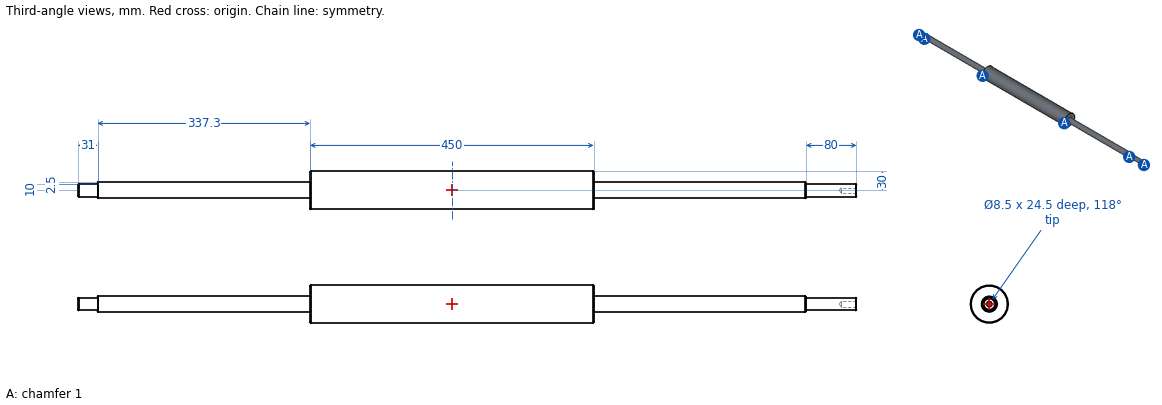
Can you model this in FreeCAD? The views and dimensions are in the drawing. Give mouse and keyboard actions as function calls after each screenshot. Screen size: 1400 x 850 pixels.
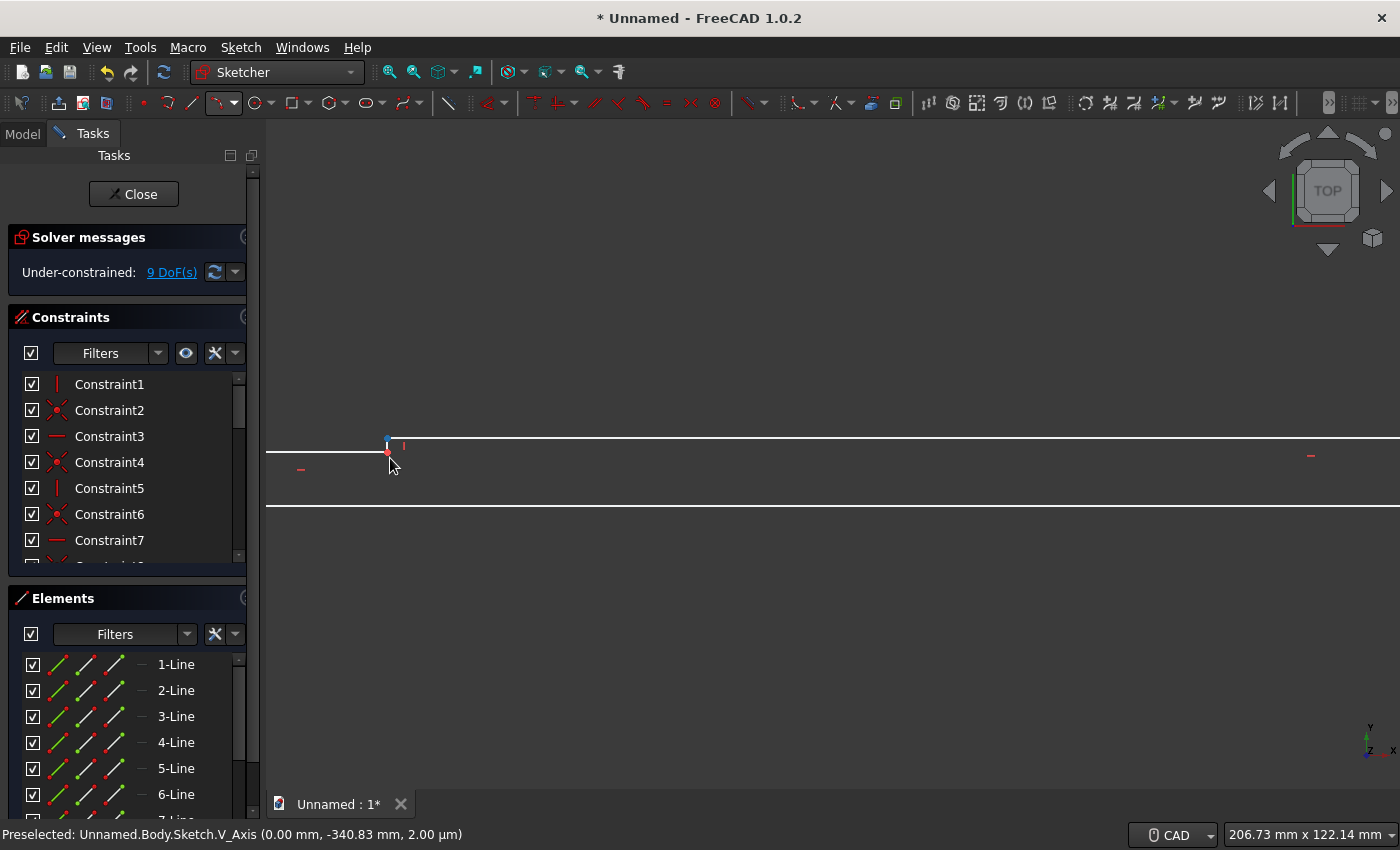
click(387, 452)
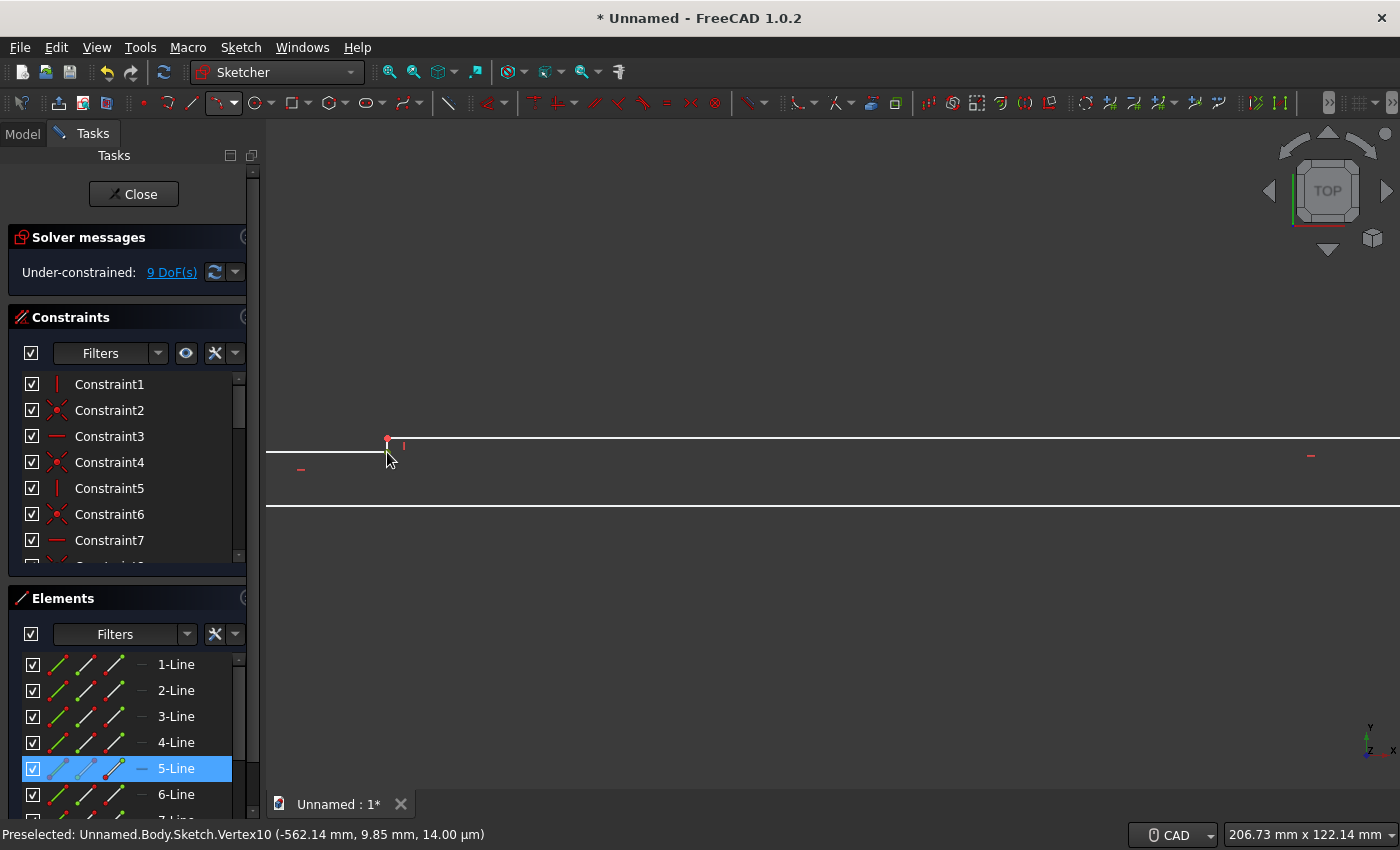
scroll(481, 457, down, 12)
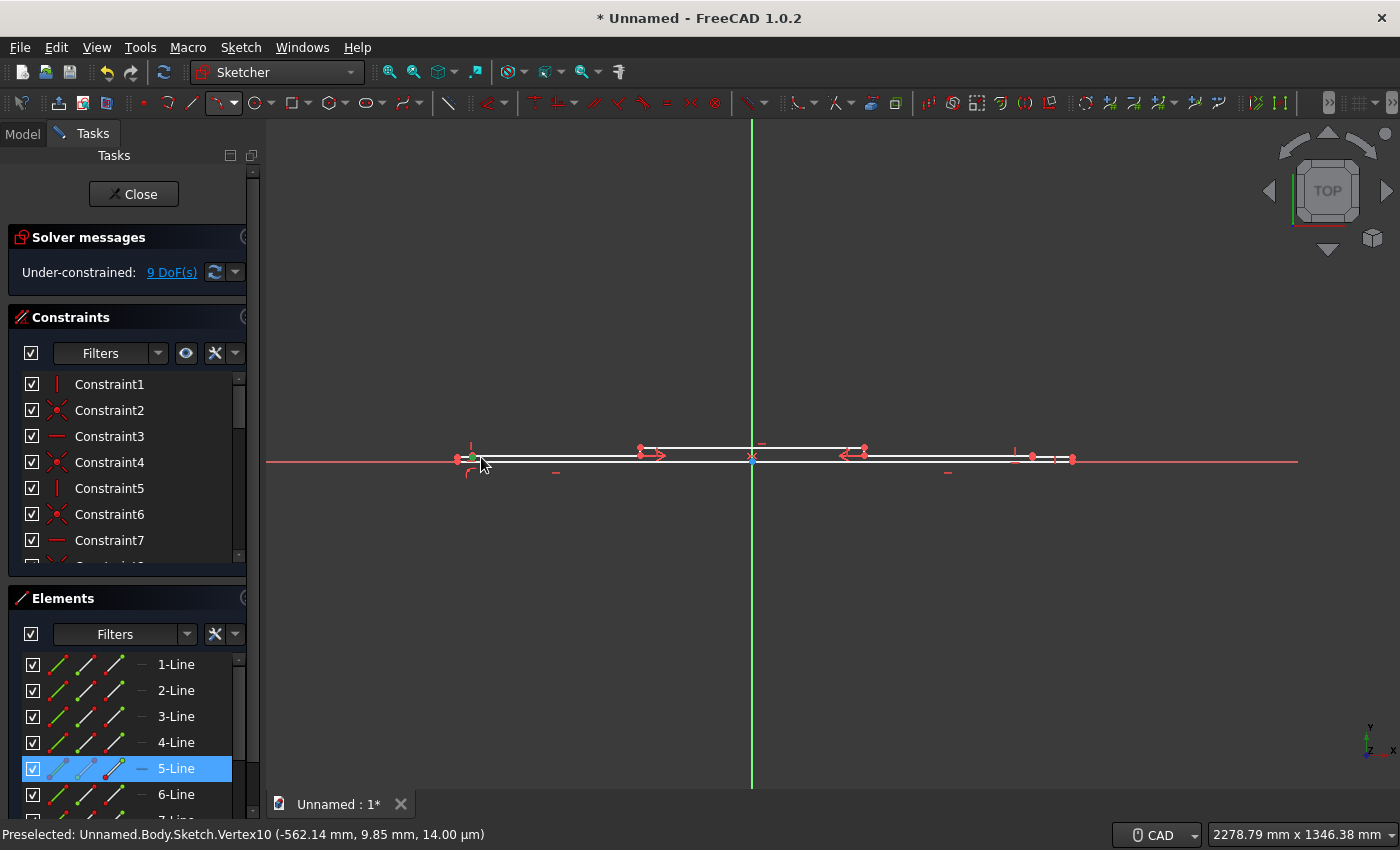
scroll(1032, 457, up, 11)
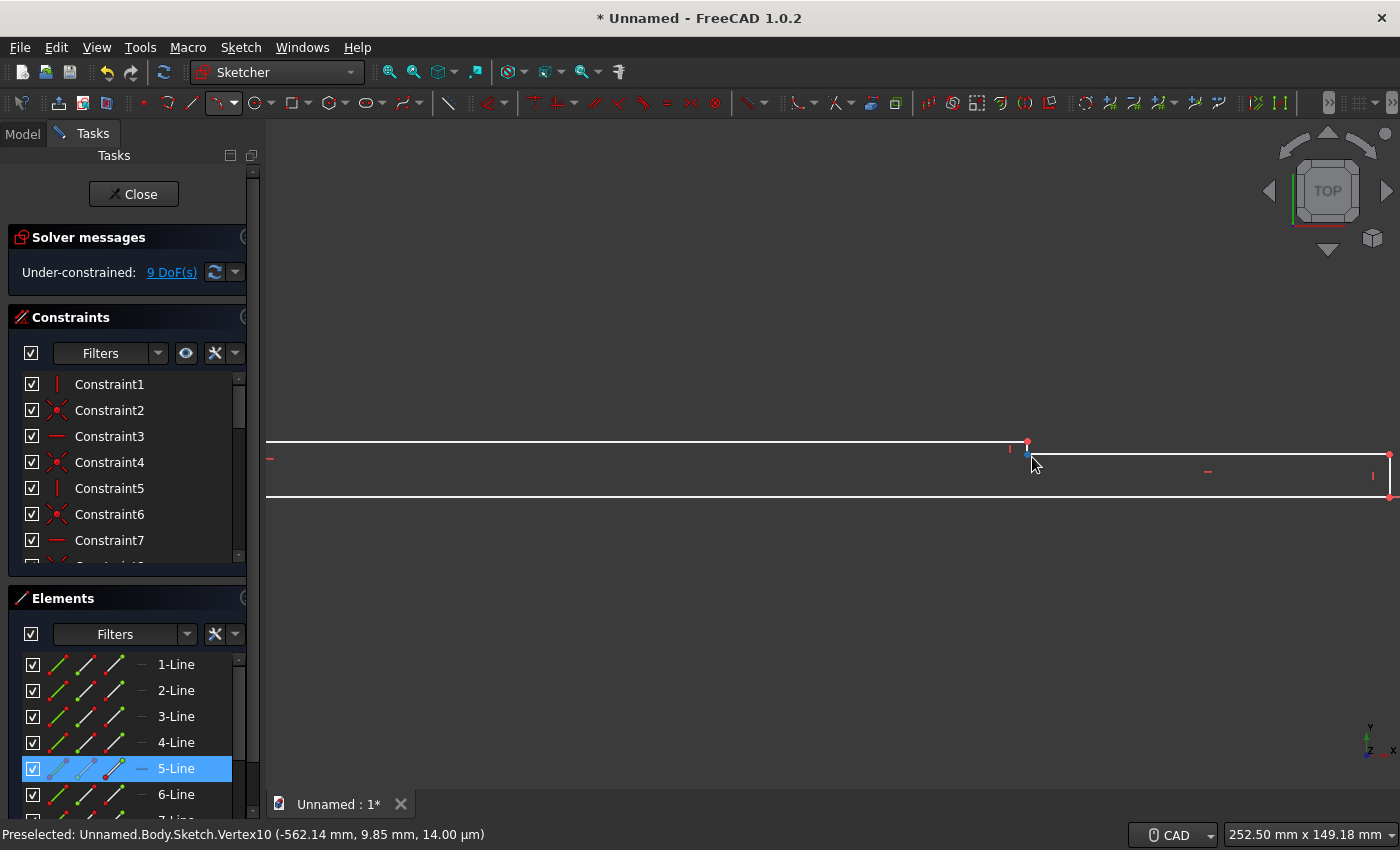
click(1027, 454)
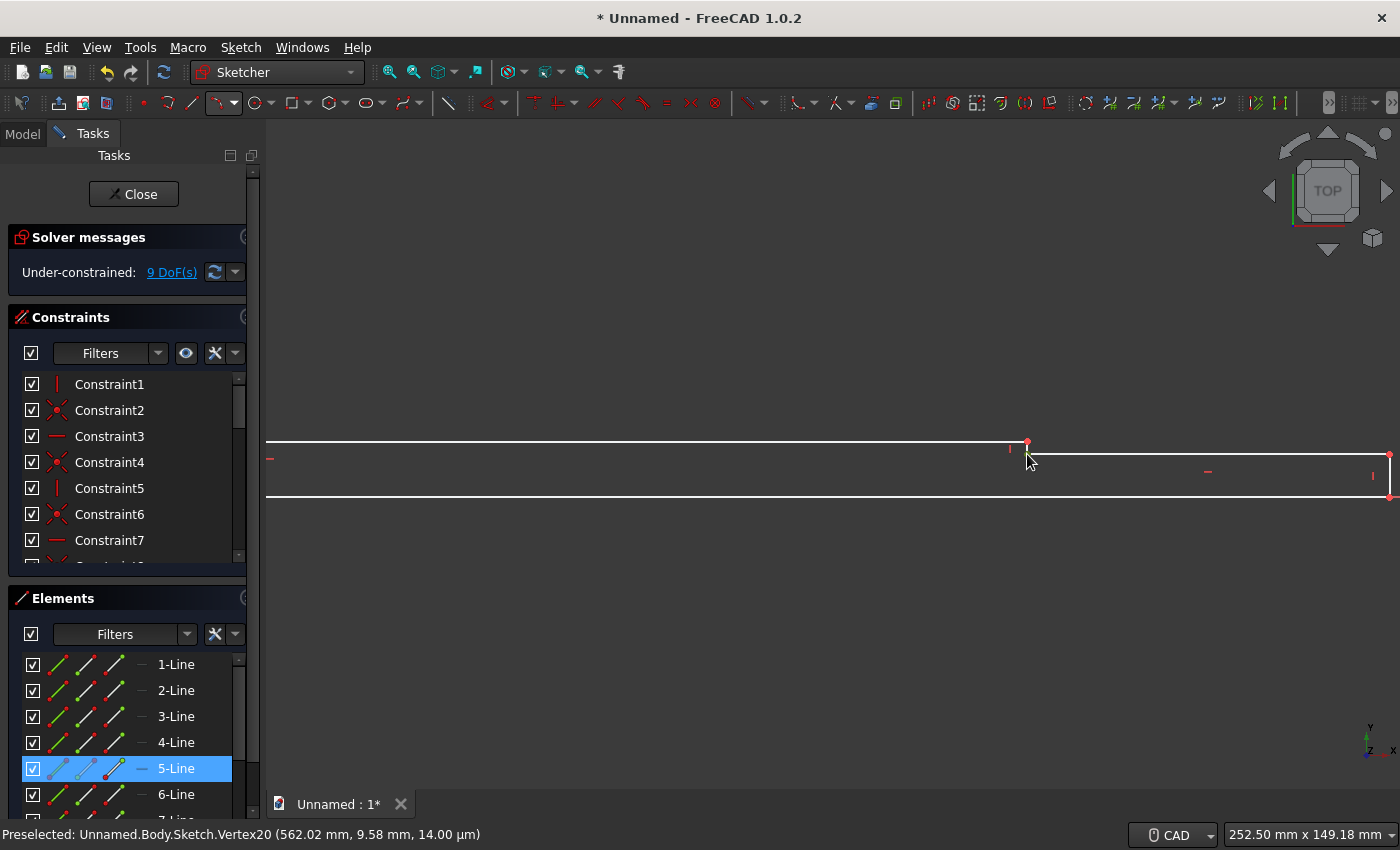
scroll(1033, 457, down, 11)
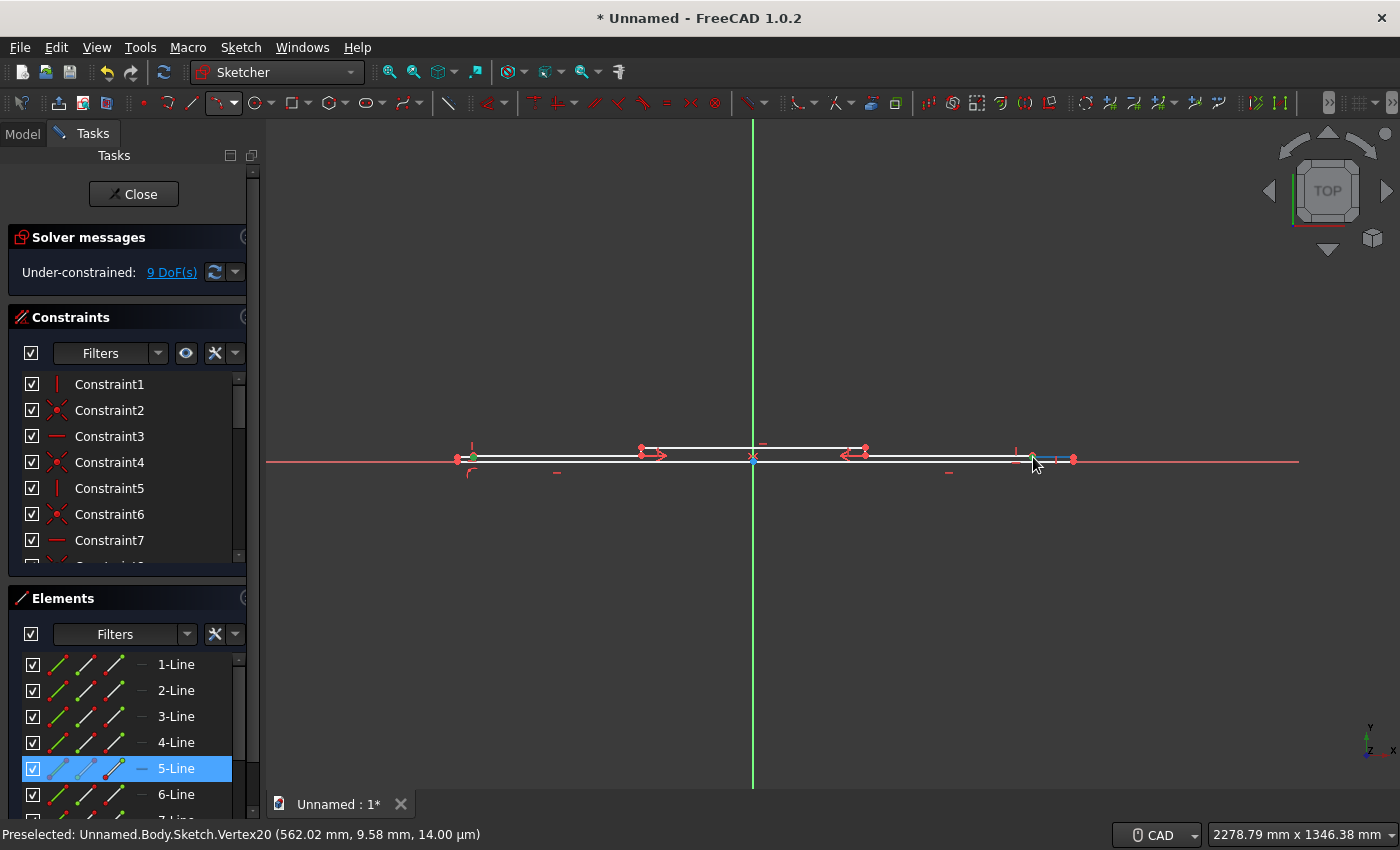
click(753, 717)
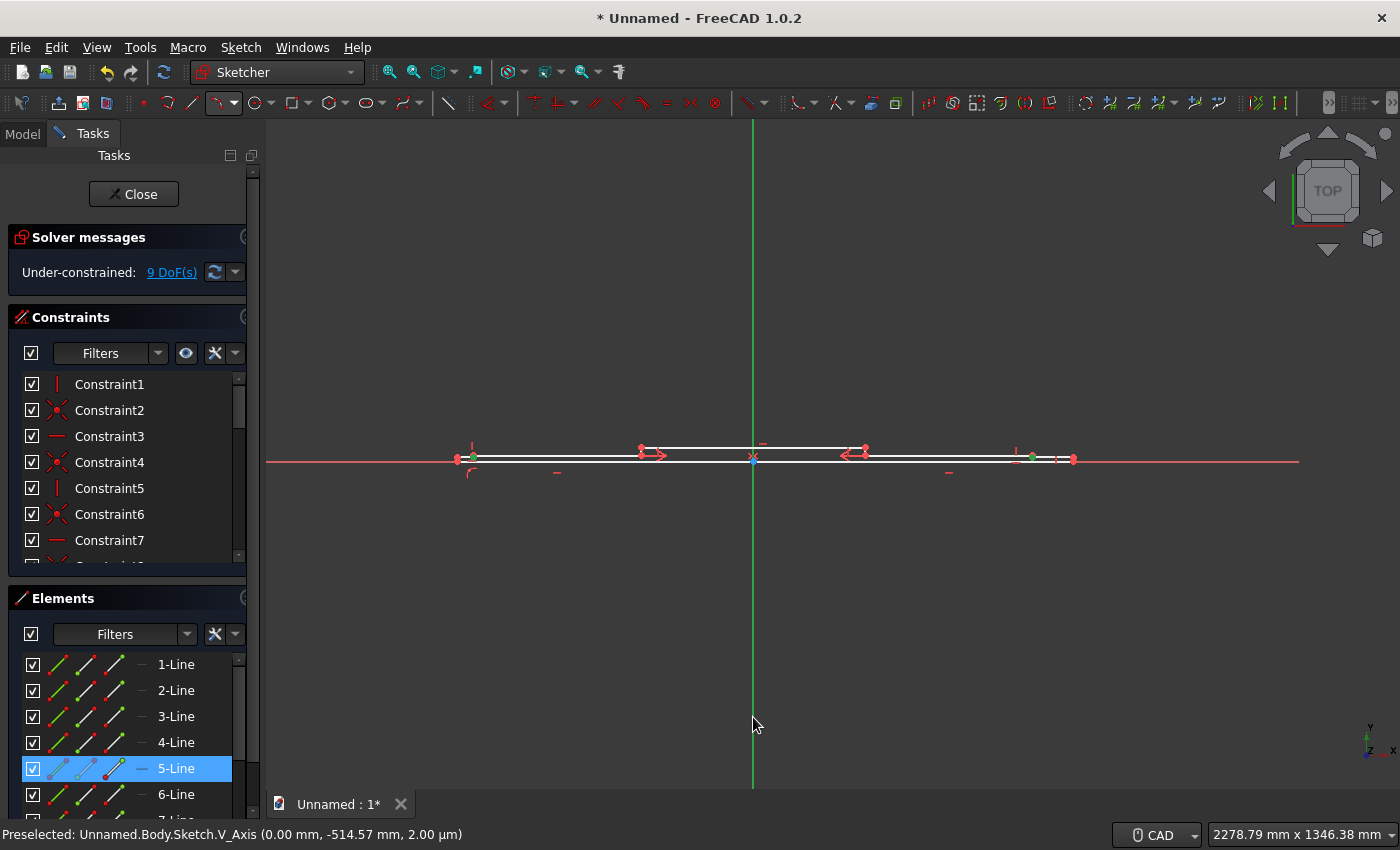
key(s)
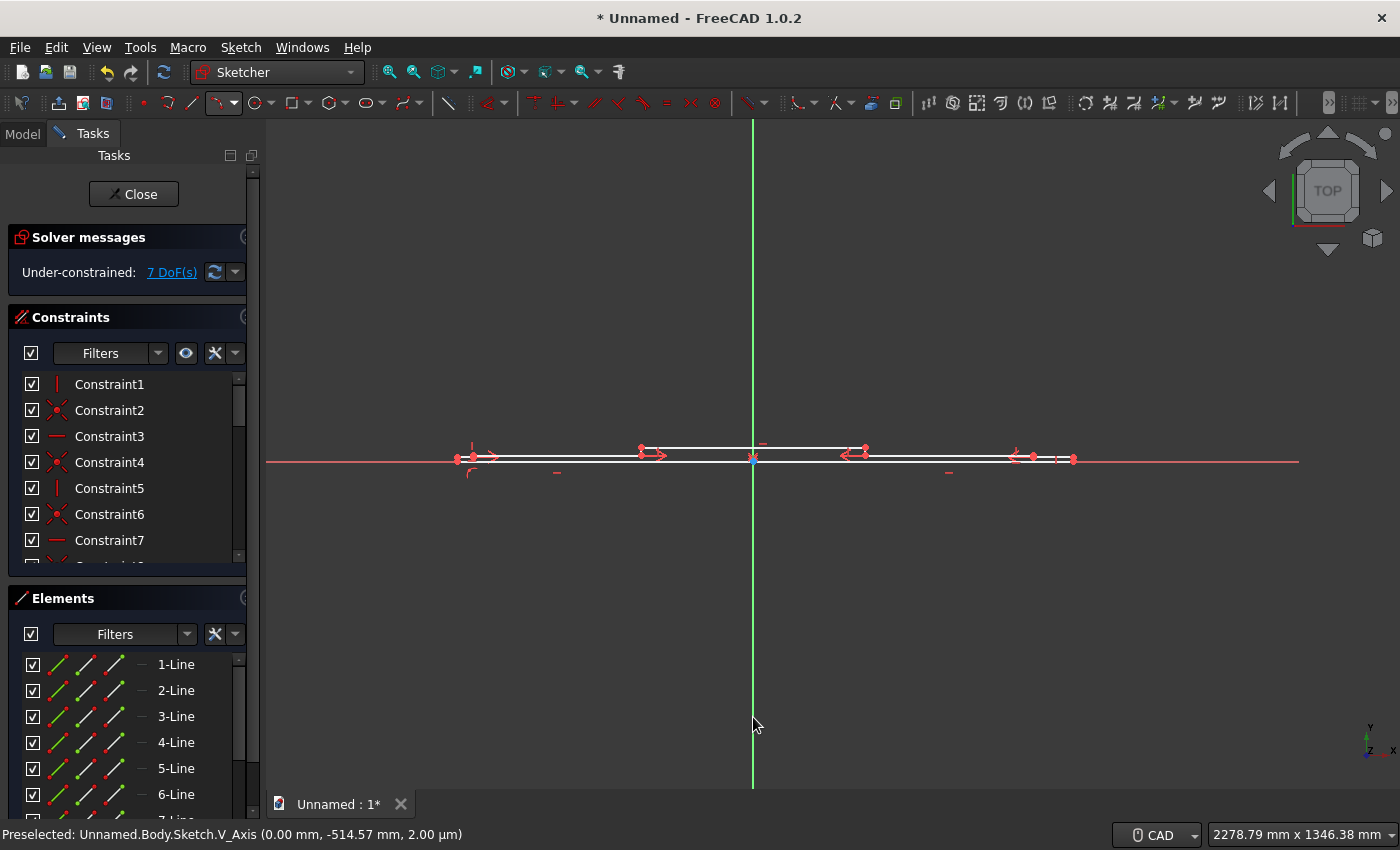
key(d)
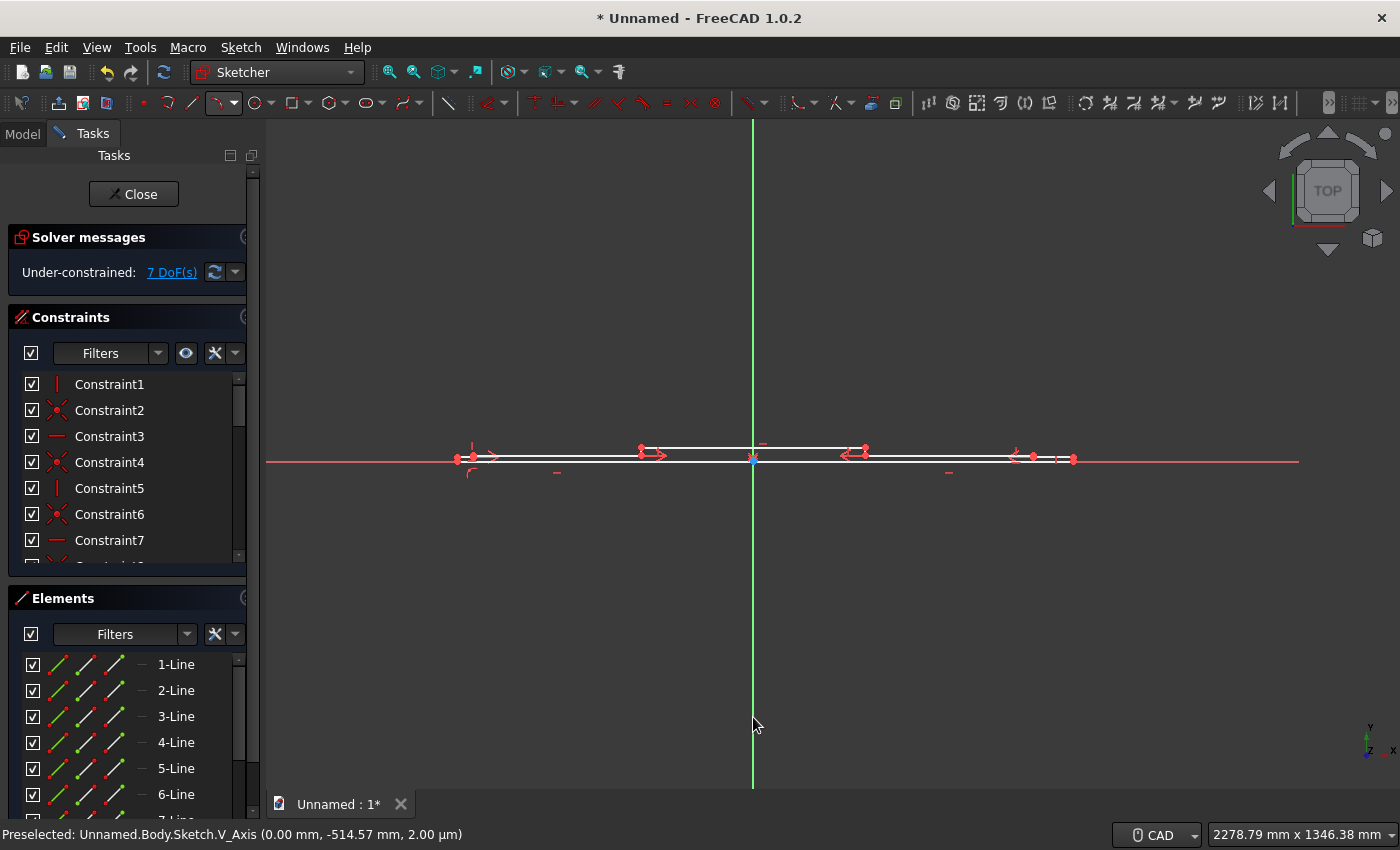
scroll(467, 457, up, 6)